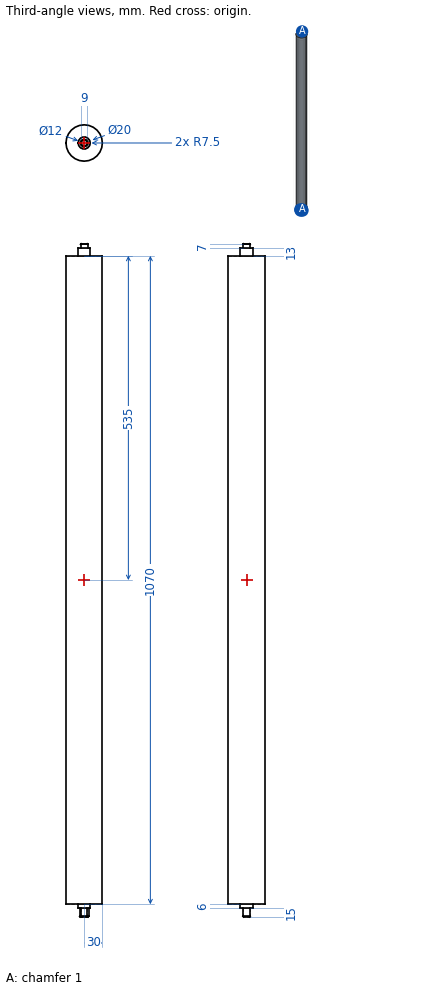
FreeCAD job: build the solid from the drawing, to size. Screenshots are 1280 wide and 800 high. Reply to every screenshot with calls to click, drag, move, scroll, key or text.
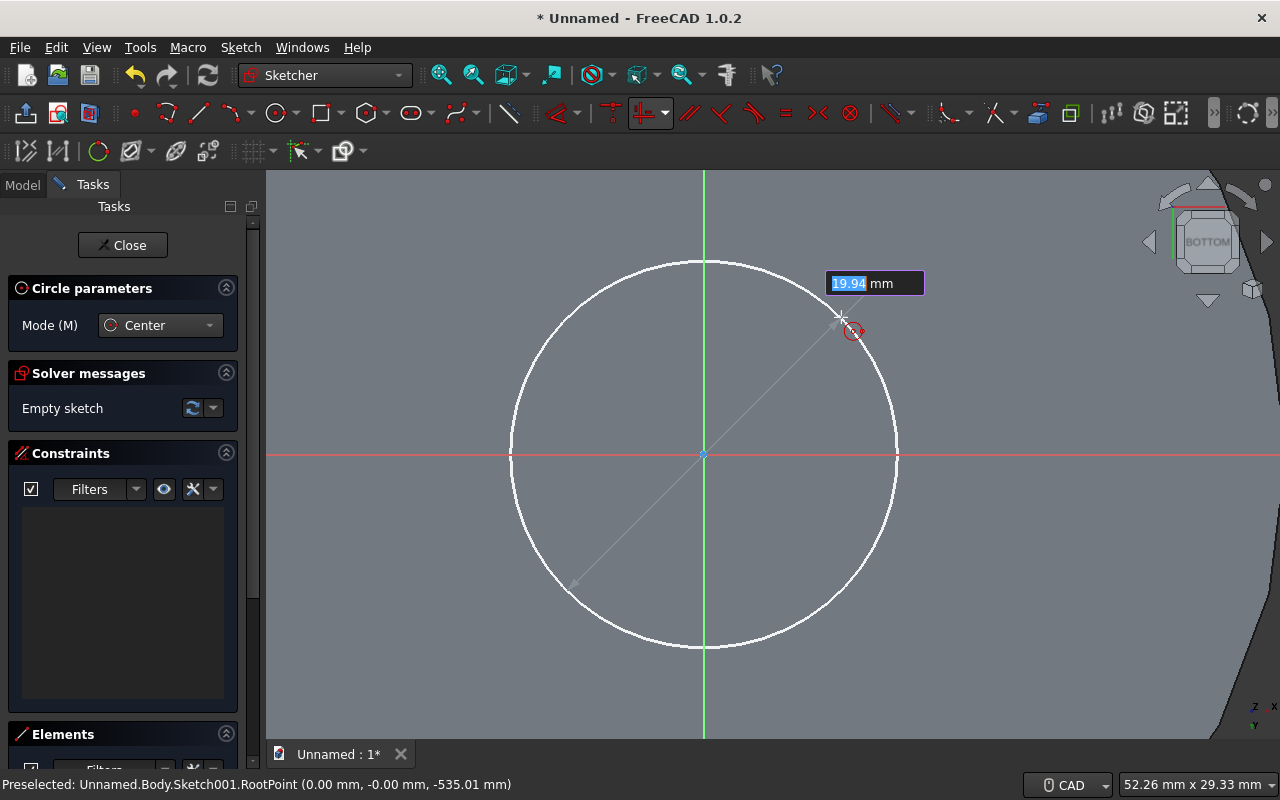
text(20)
key(Return)
key(Escape)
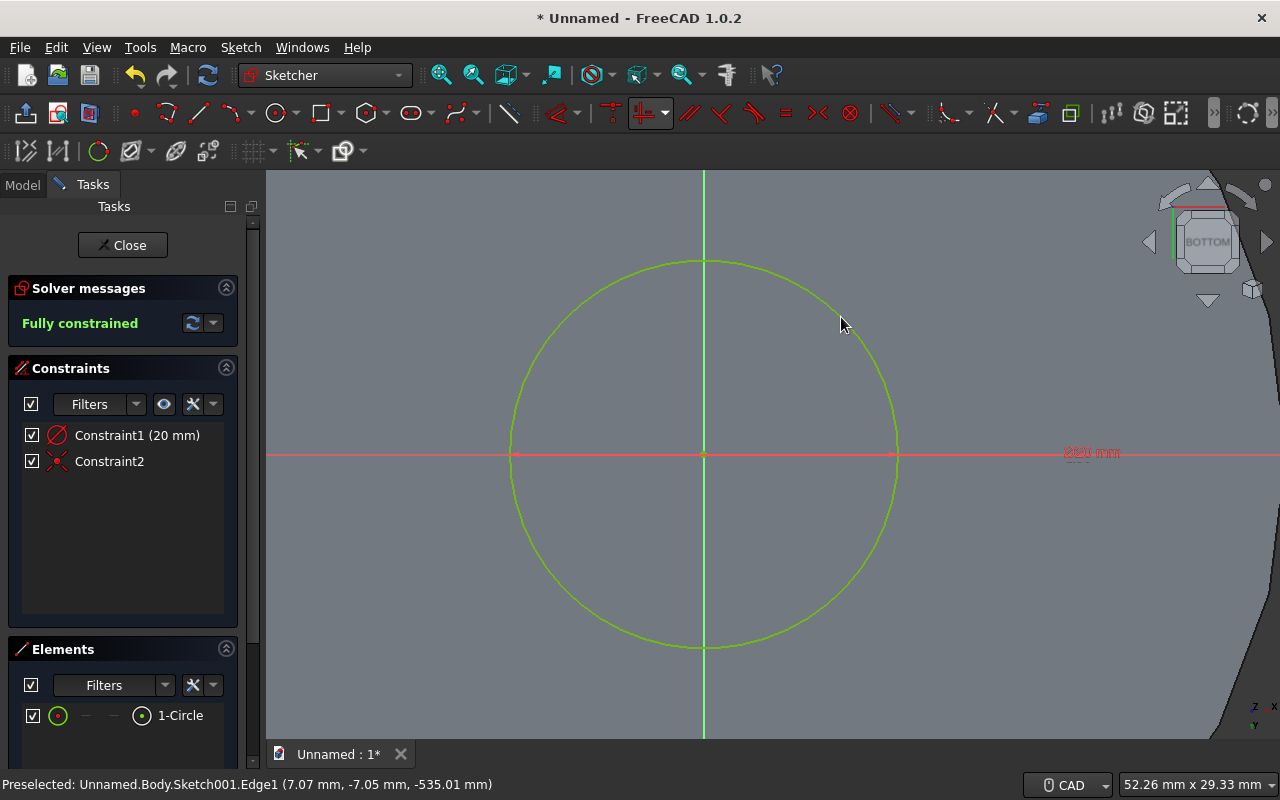
click(123, 245)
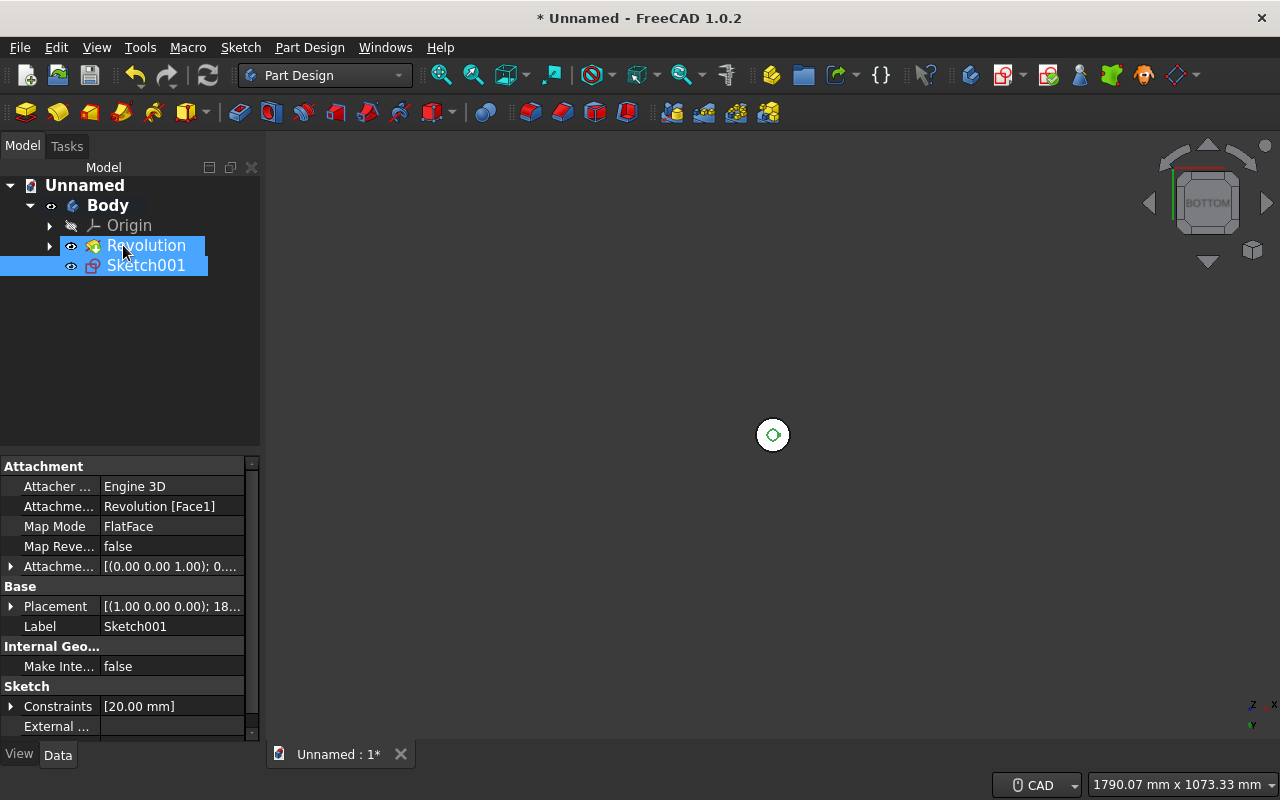
click(26, 112)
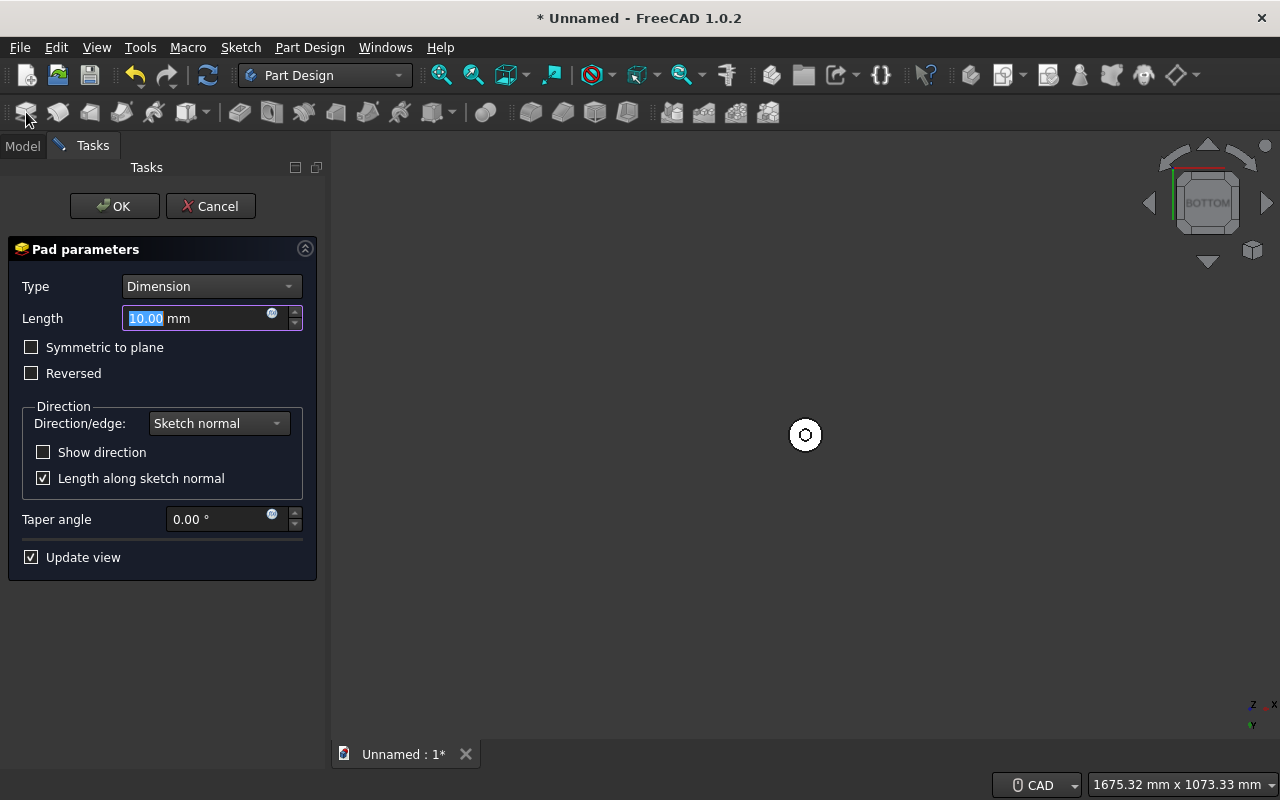
text(6)
key(Tab)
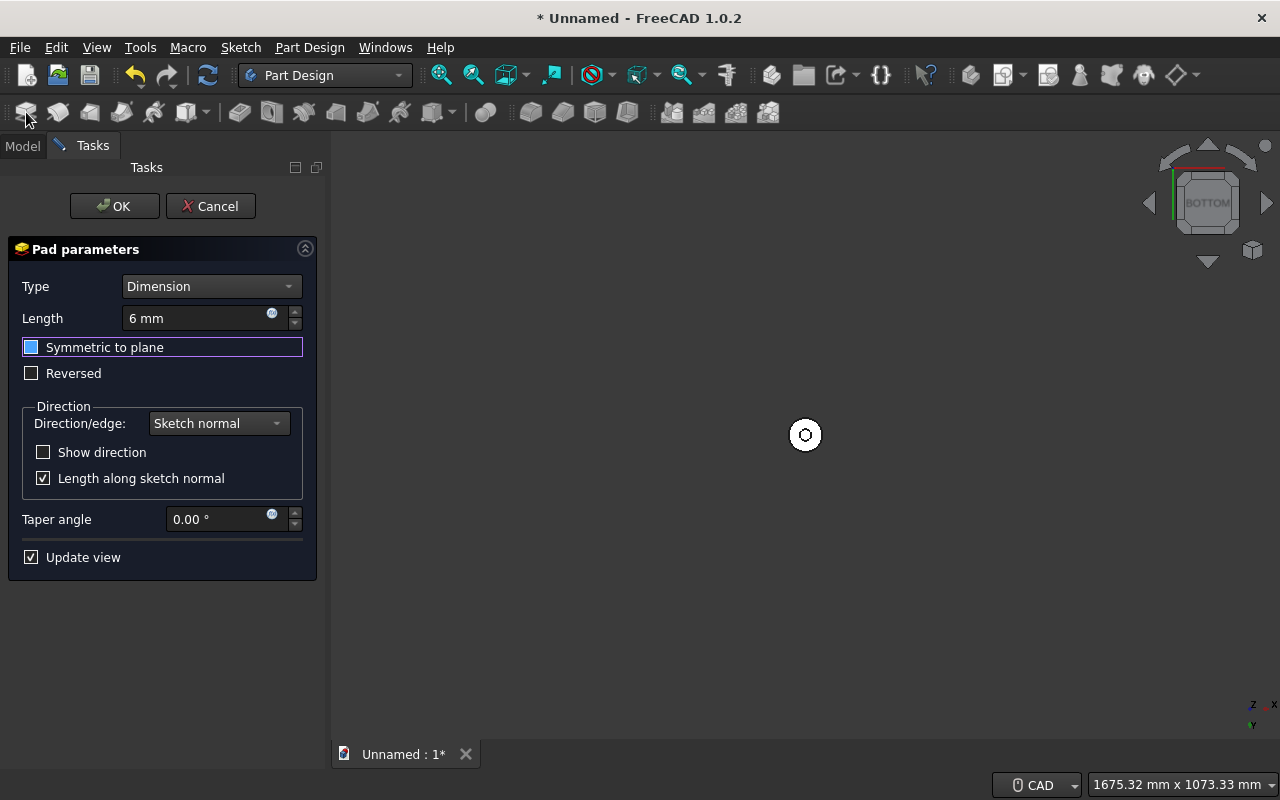
click(115, 206)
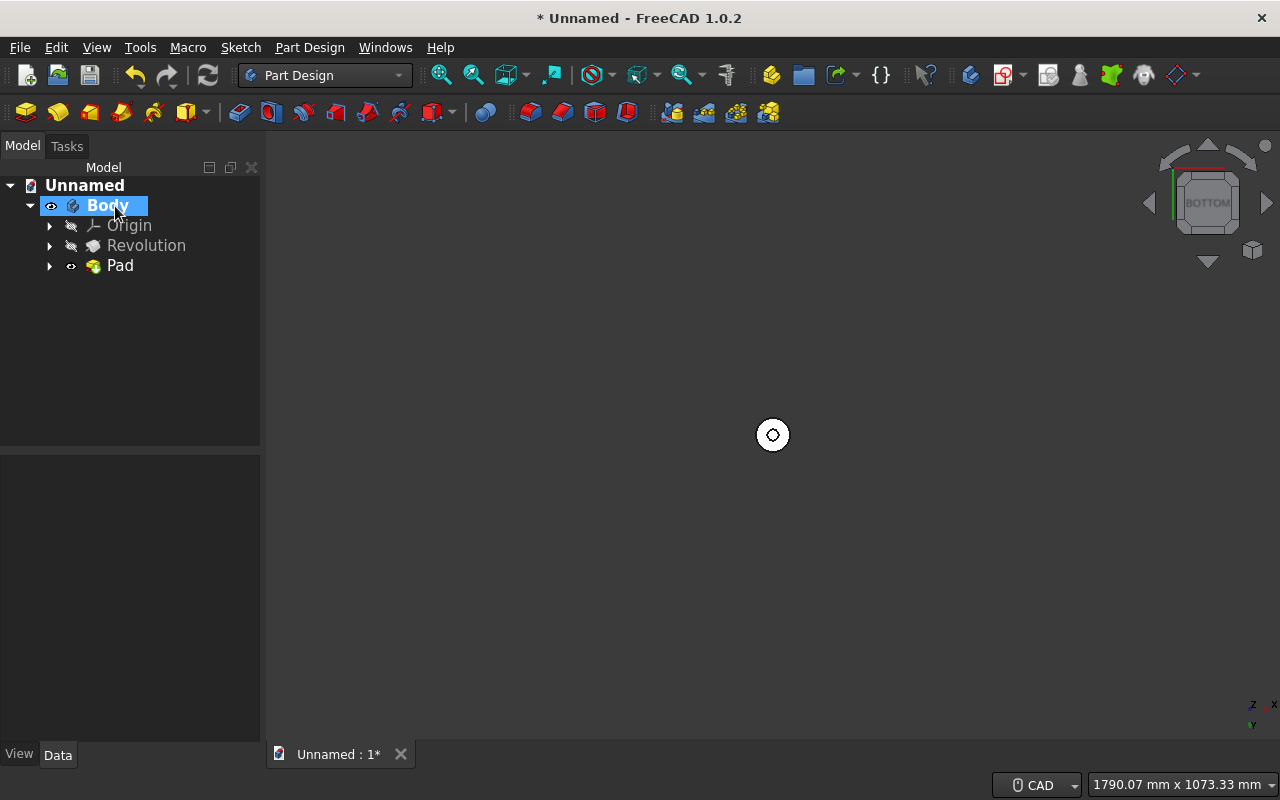
key(v)
key(f)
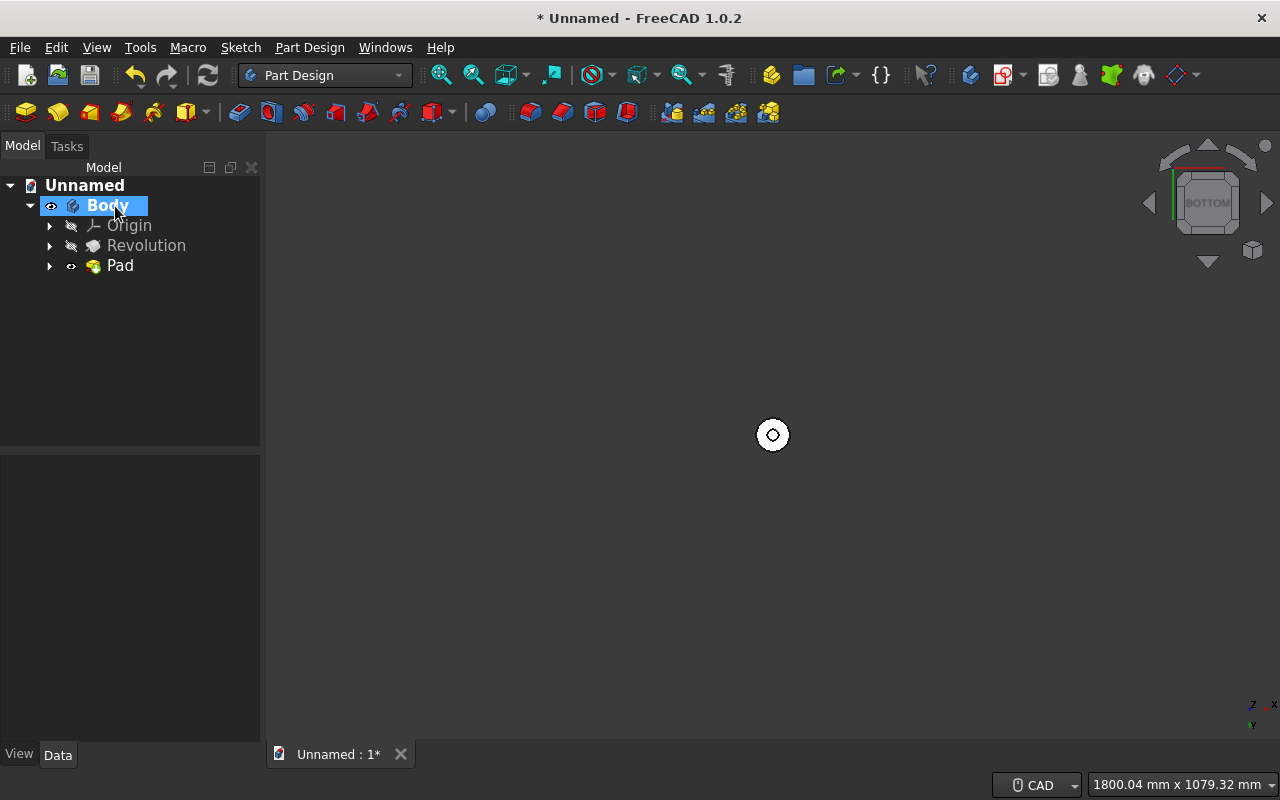
scroll(773, 434, up, 4)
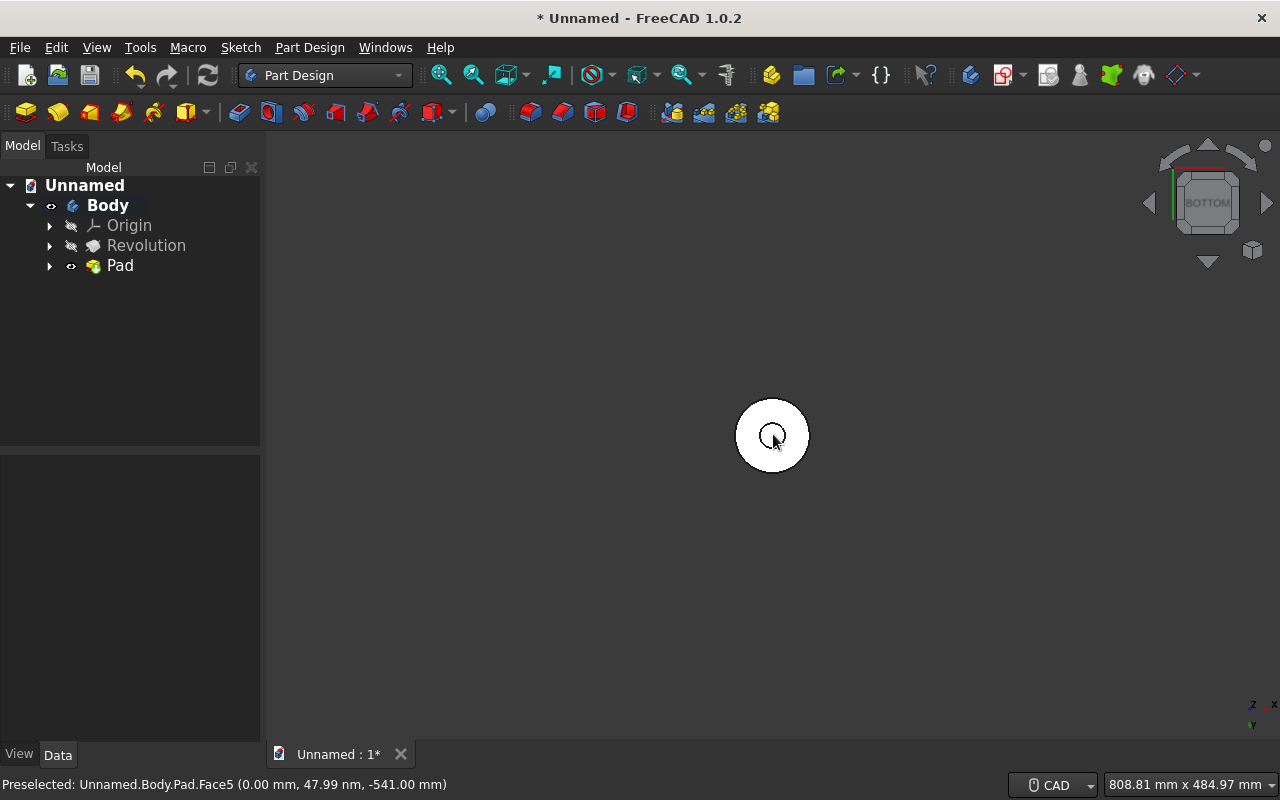
click(772, 435)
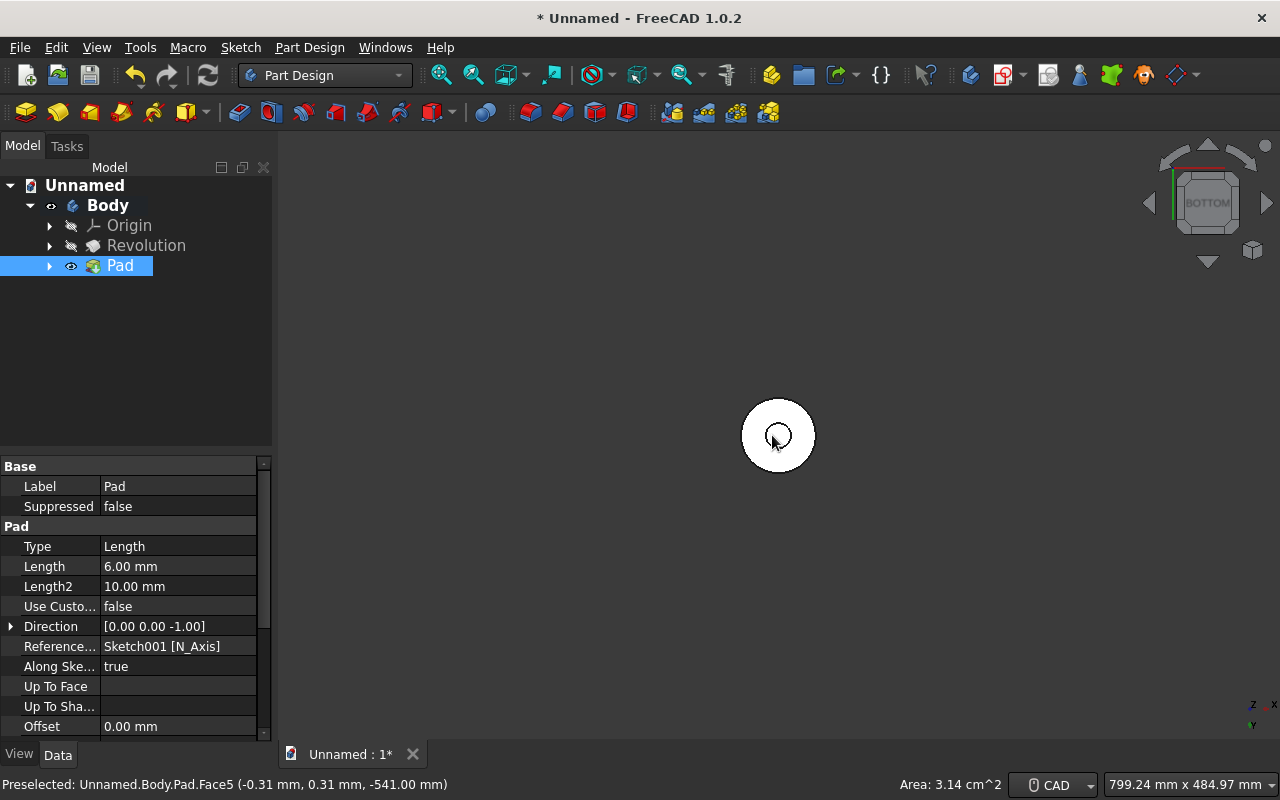
click(1004, 76)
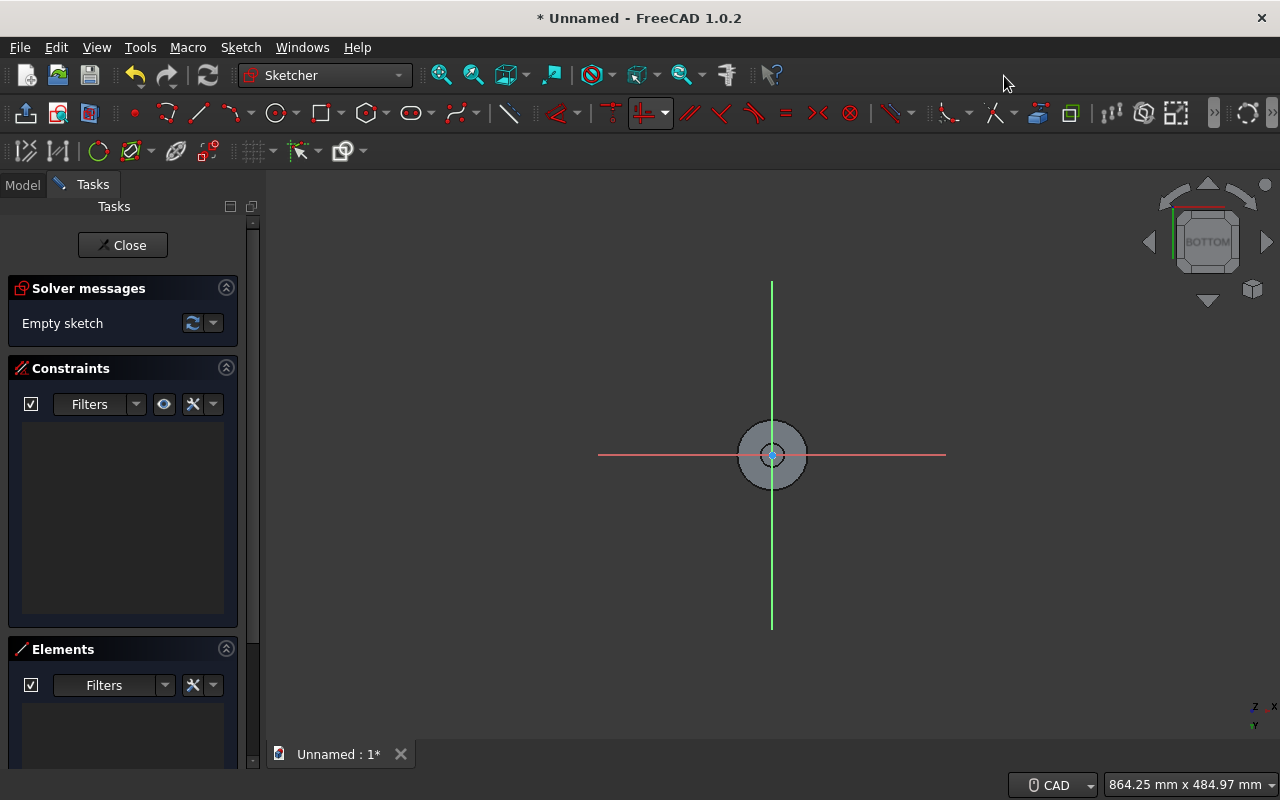
scroll(776, 455, up, 15)